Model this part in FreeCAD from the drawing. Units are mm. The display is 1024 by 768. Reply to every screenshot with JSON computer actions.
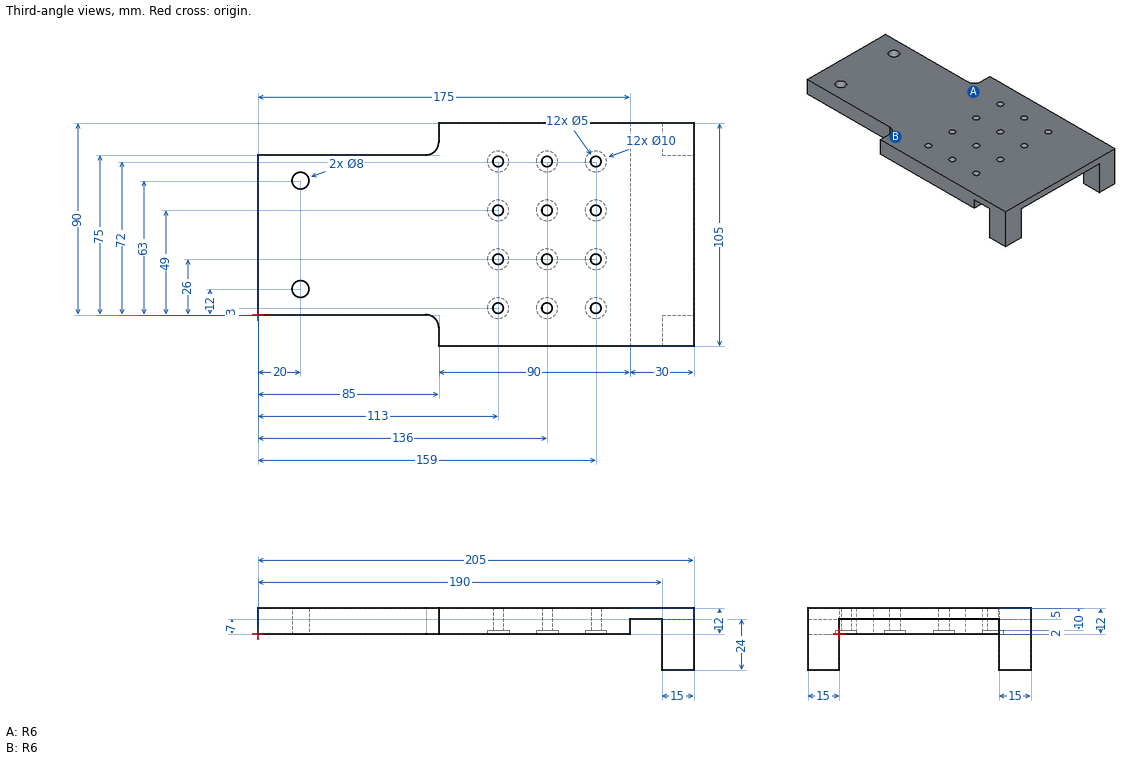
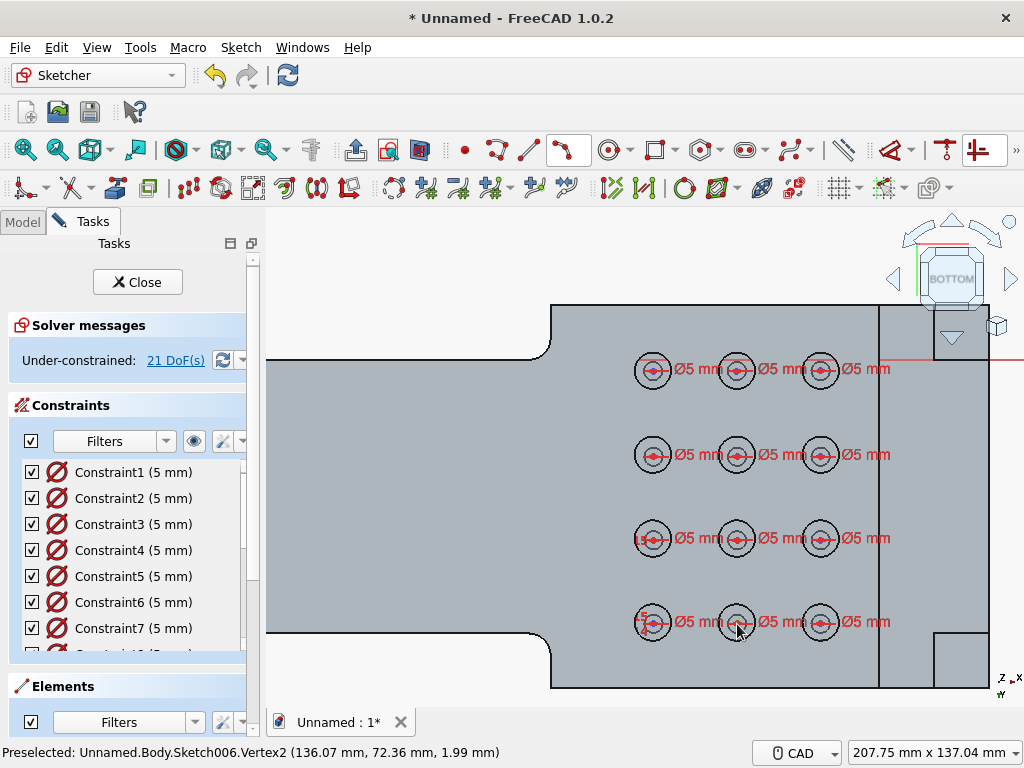
{"action": "left_click", "coordinate": [737, 540]}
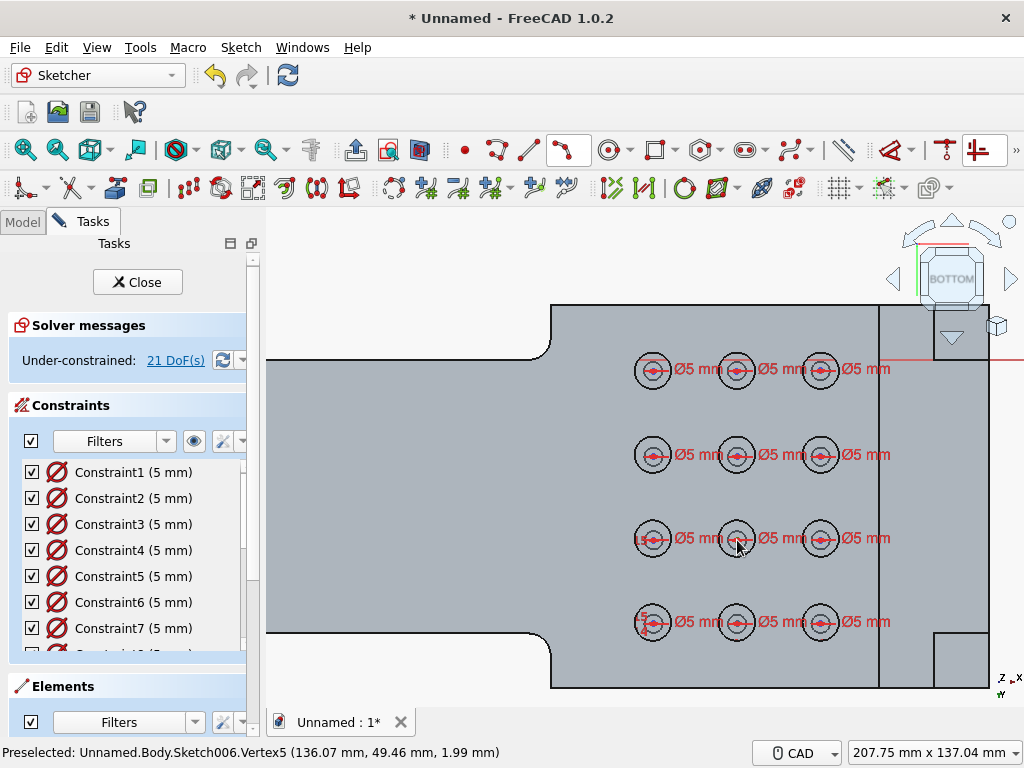
{"action": "key", "text": "v"}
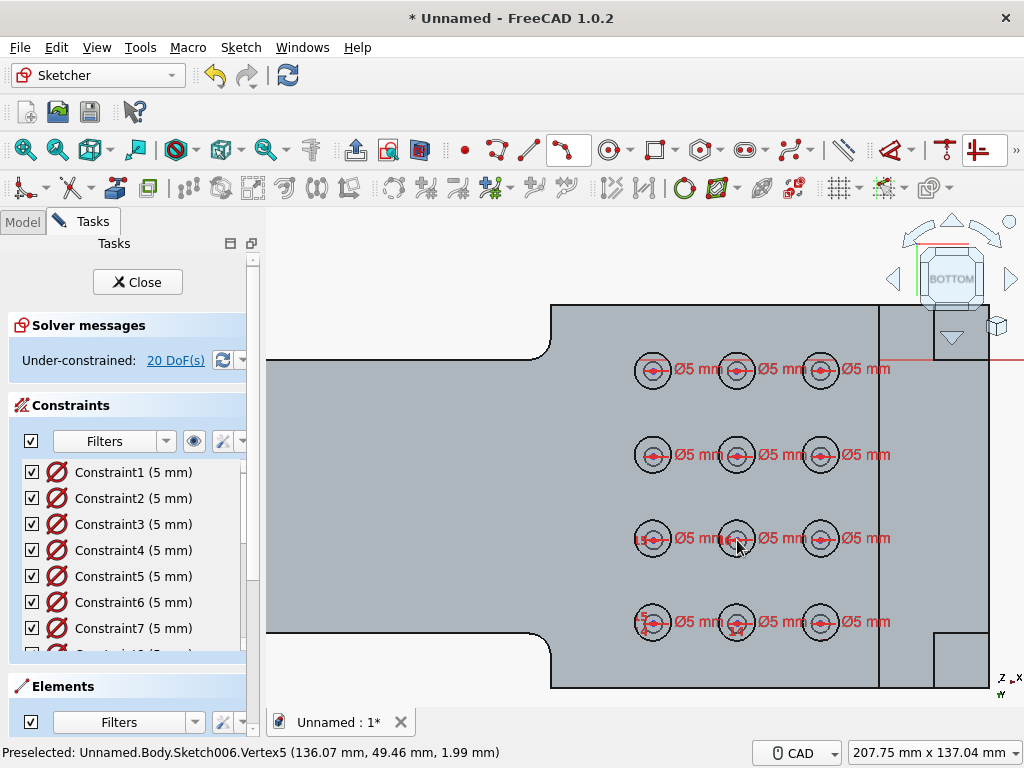
{"action": "left_click", "coordinate": [654, 540]}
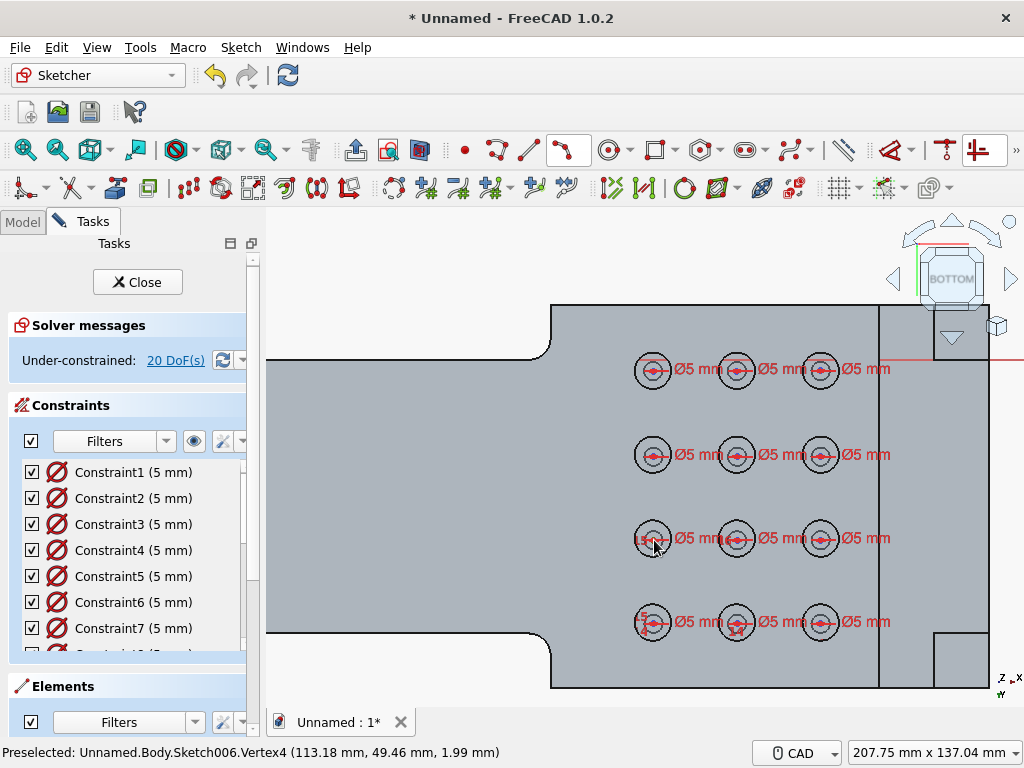
{"action": "left_click", "coordinate": [737, 540]}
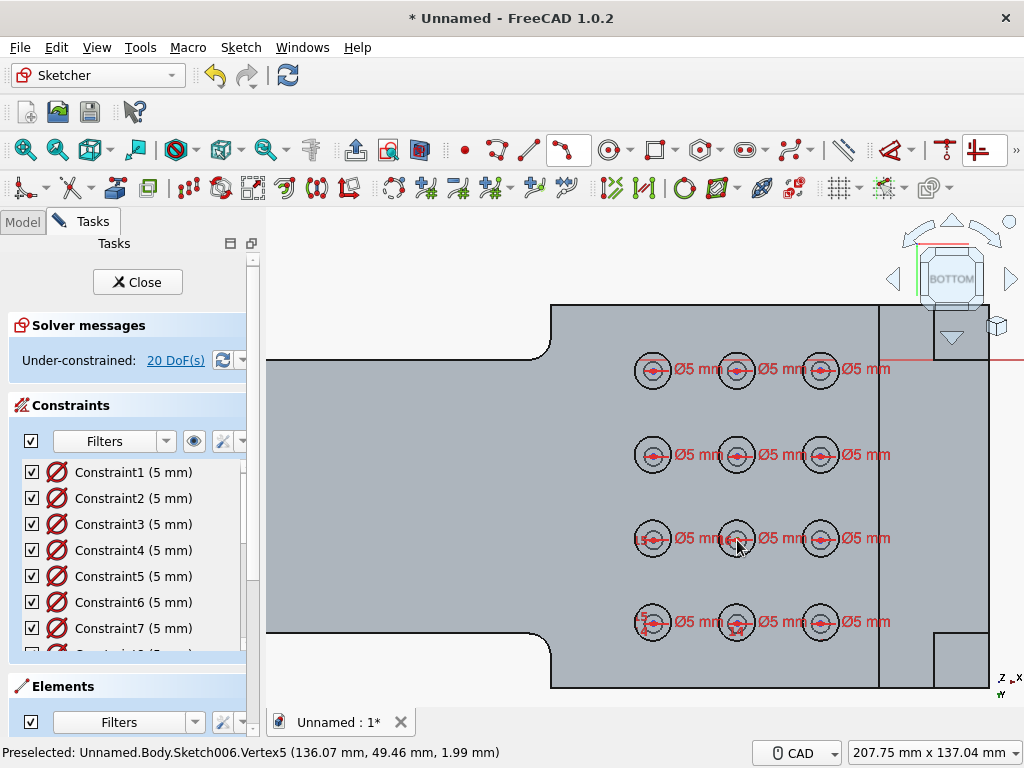
{"action": "key", "text": "h"}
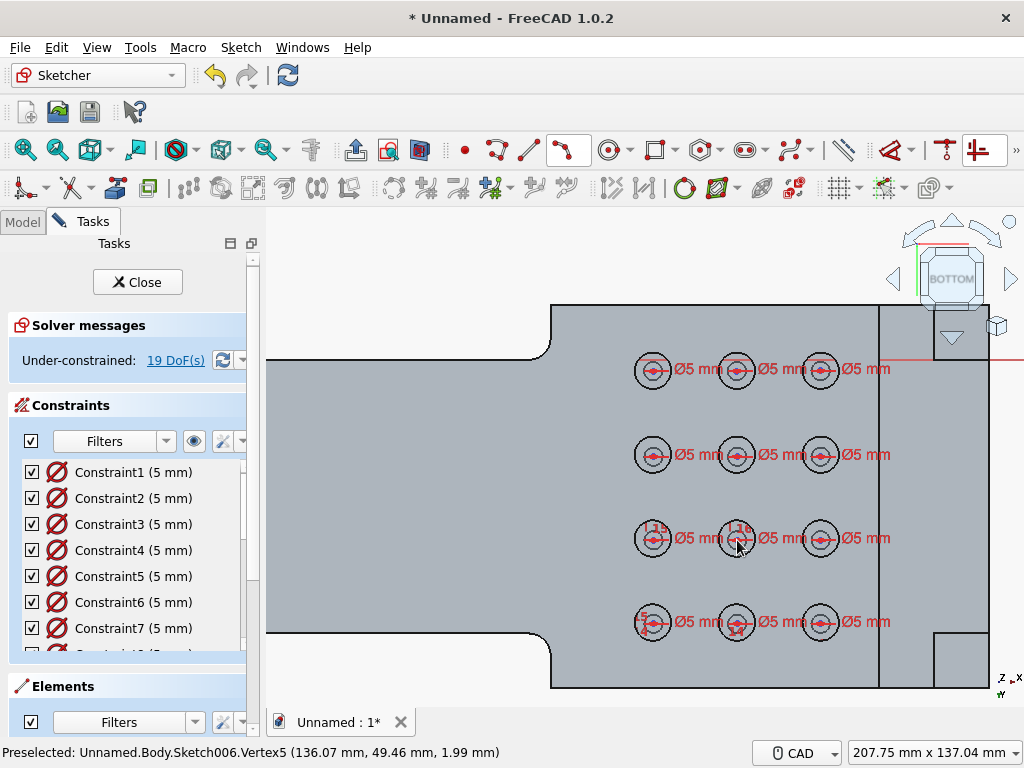
{"action": "left_click", "coordinate": [821, 624]}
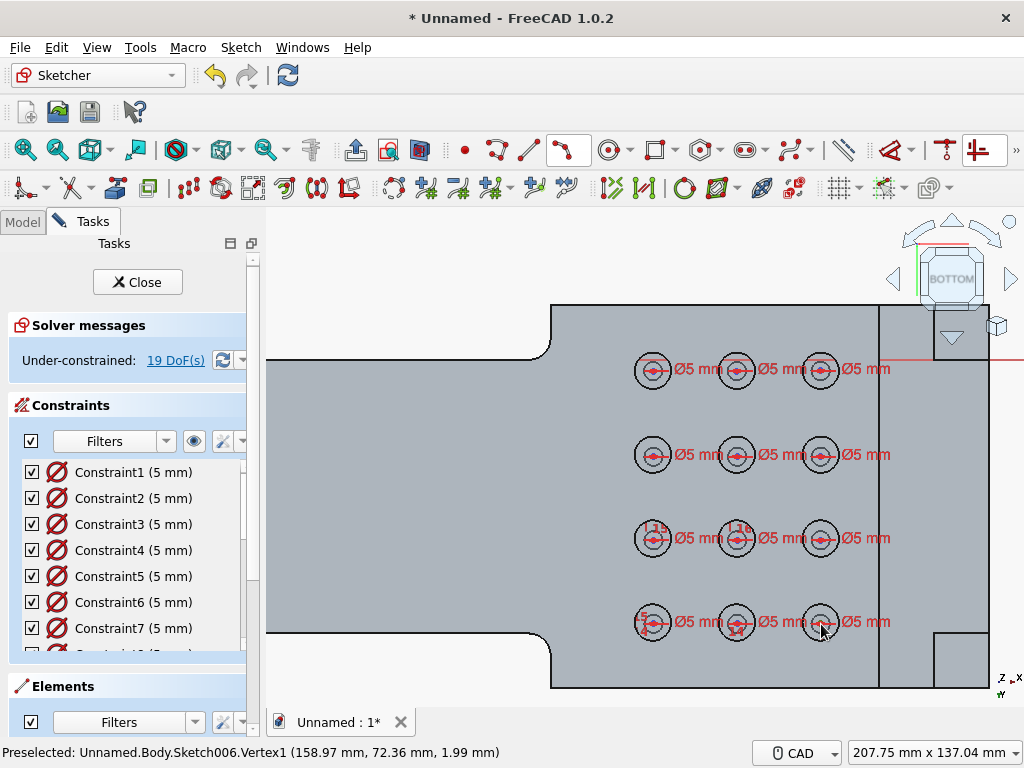
{"action": "left_click", "coordinate": [821, 540]}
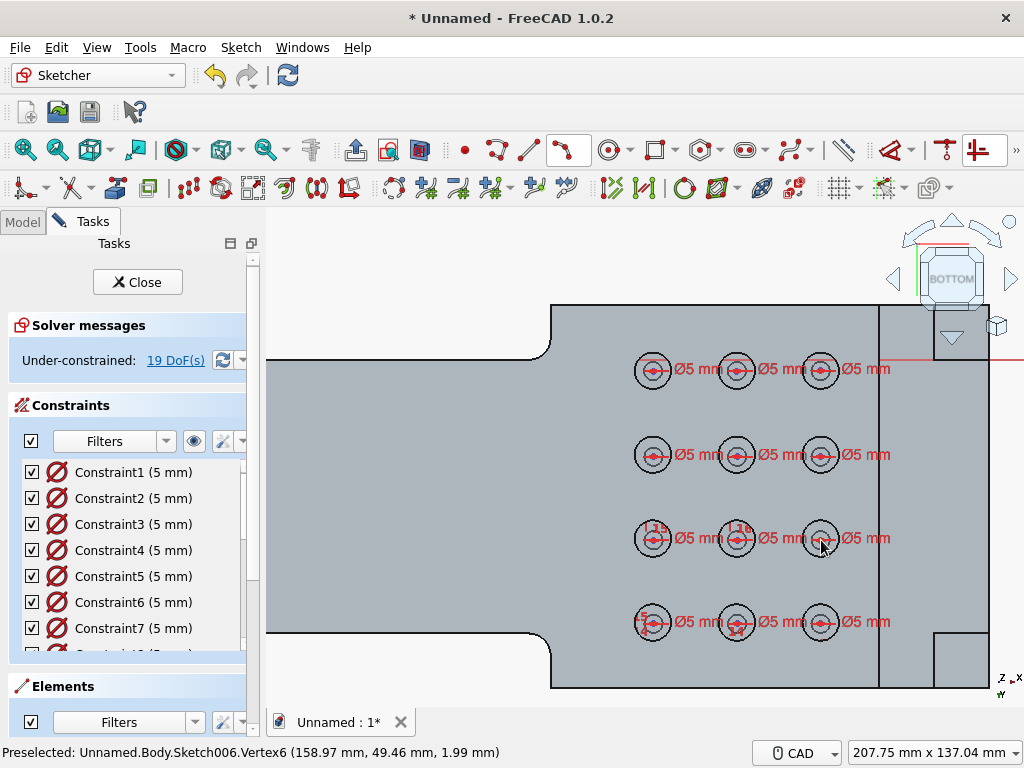
{"action": "key", "text": "v"}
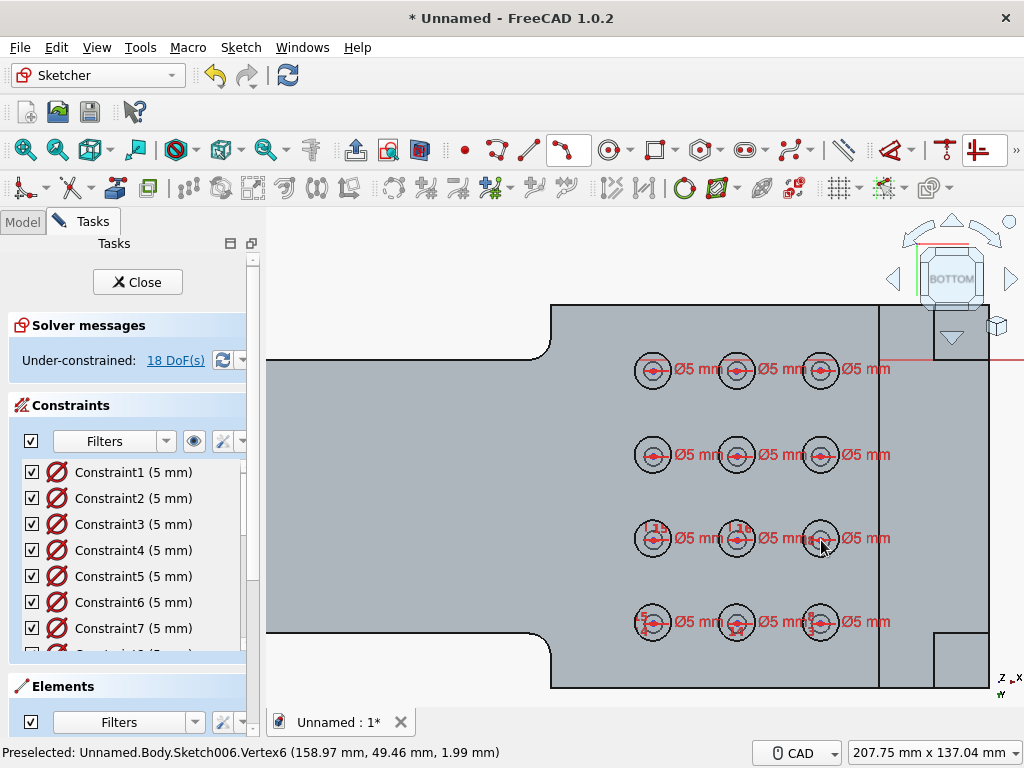
{"action": "left_click", "coordinate": [737, 540]}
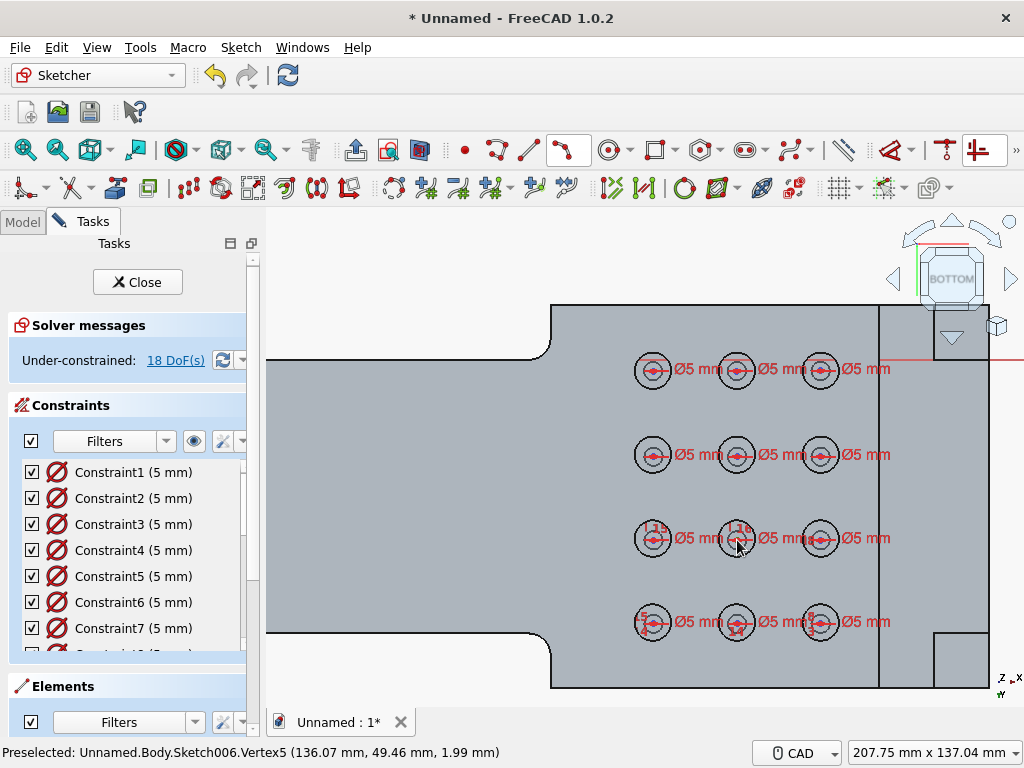
{"action": "left_click", "coordinate": [821, 540]}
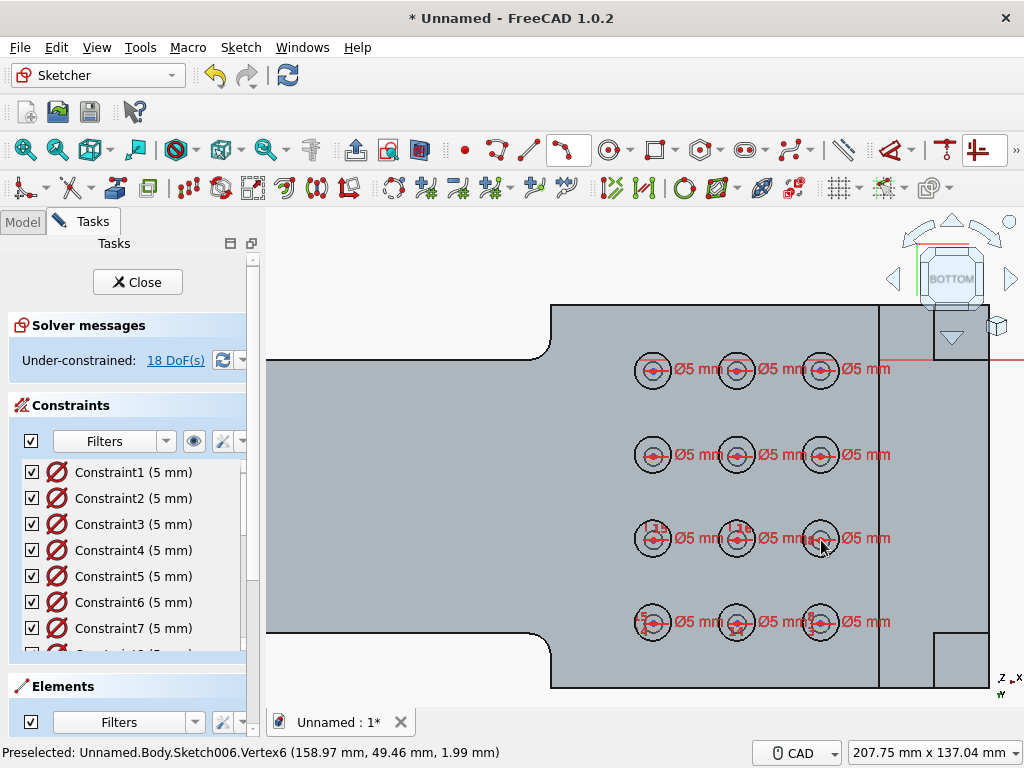
{"action": "left_click", "coordinate": [1002, 150]}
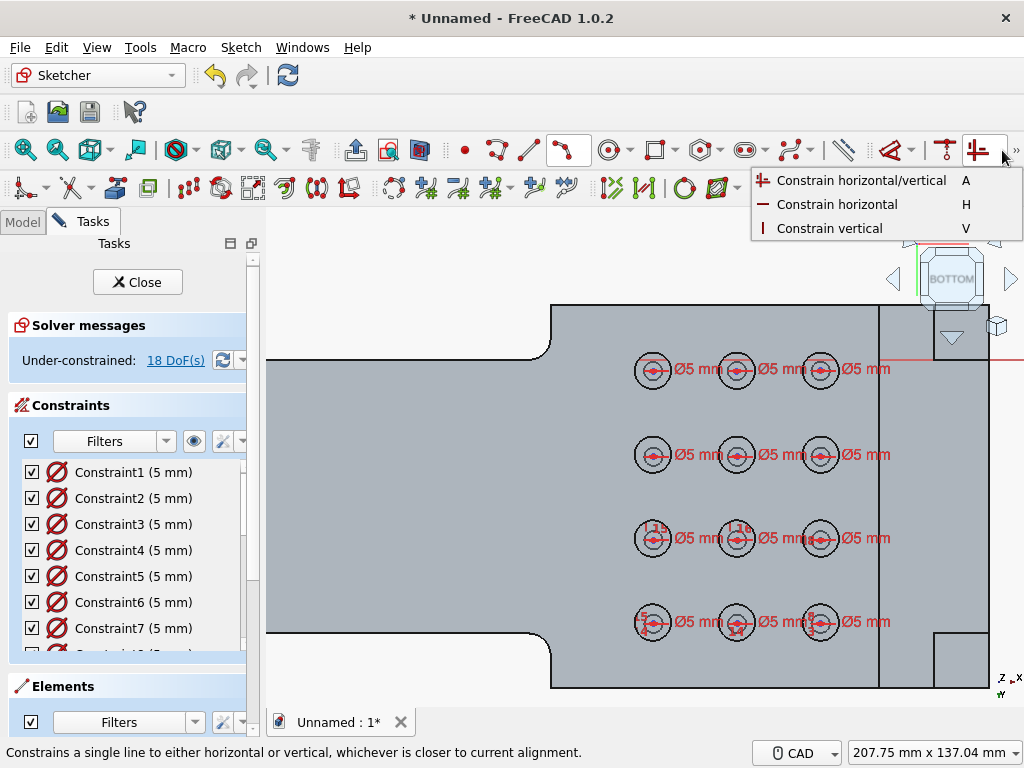
{"action": "left_click", "coordinate": [887, 204]}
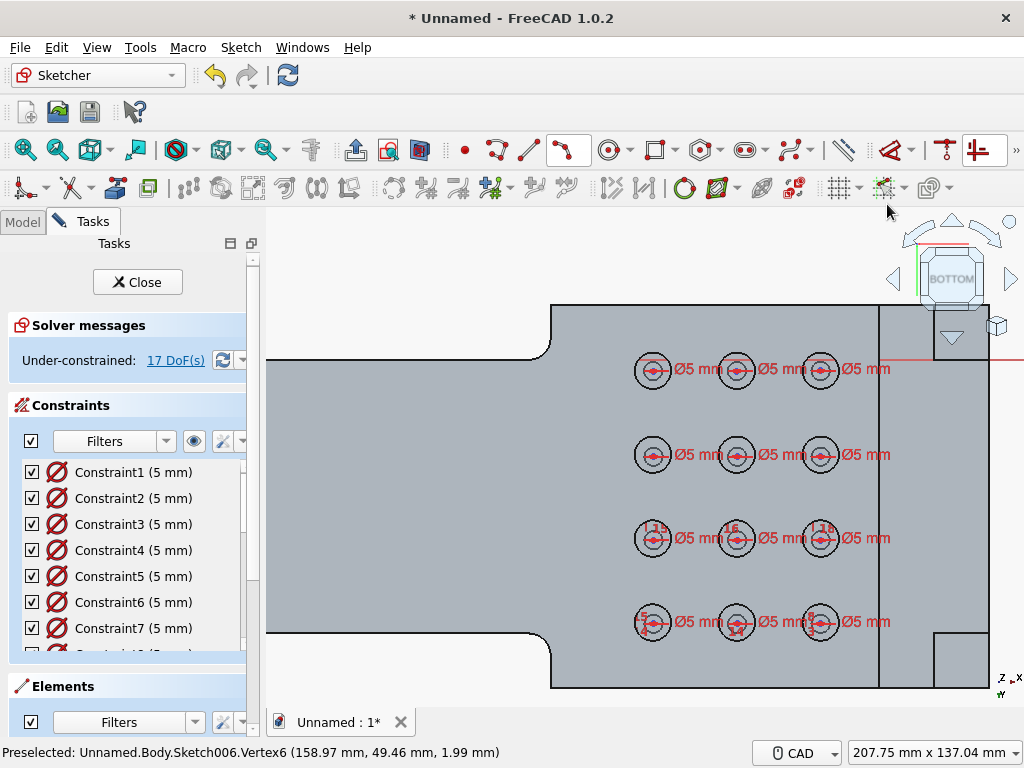
{"action": "left_click", "coordinate": [821, 540]}